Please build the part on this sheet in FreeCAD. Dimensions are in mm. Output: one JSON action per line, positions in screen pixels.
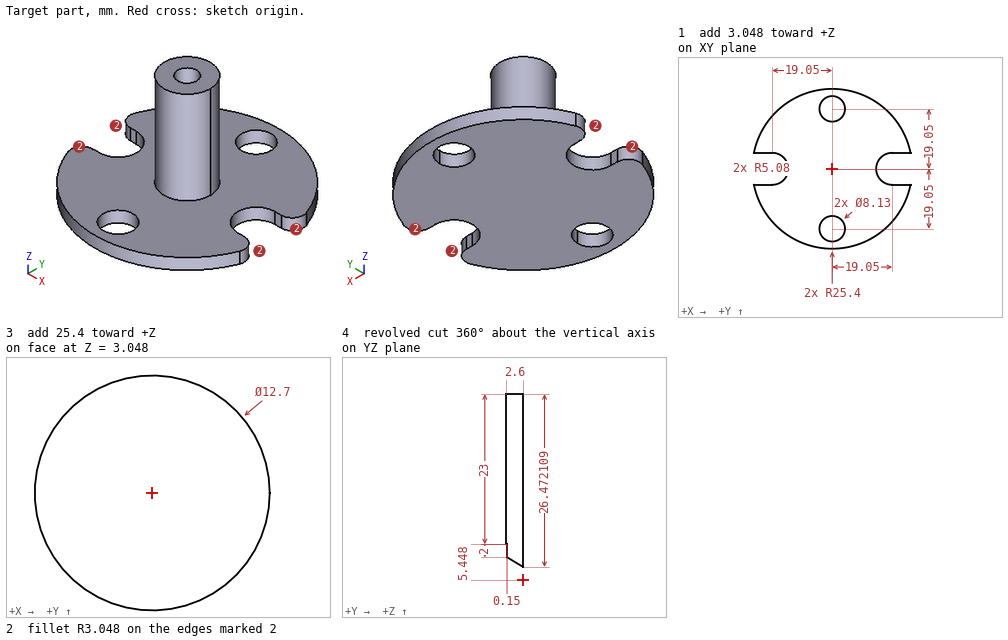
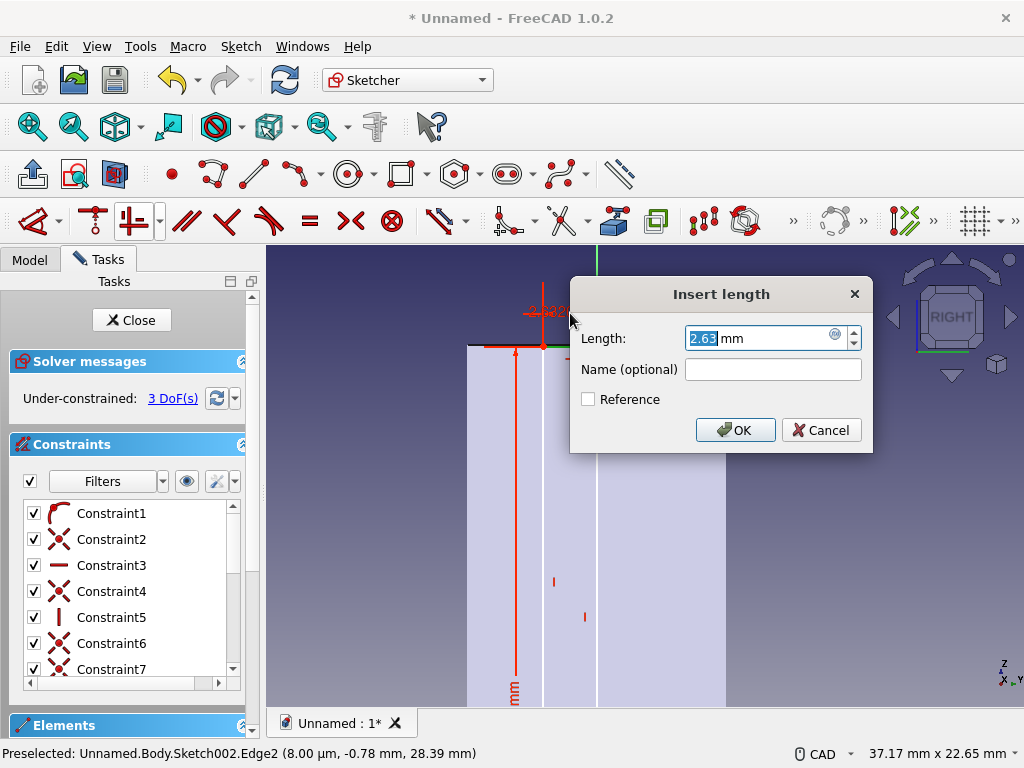
{"action": "type", "text": "2.6"}
{"action": "key", "text": "Return"}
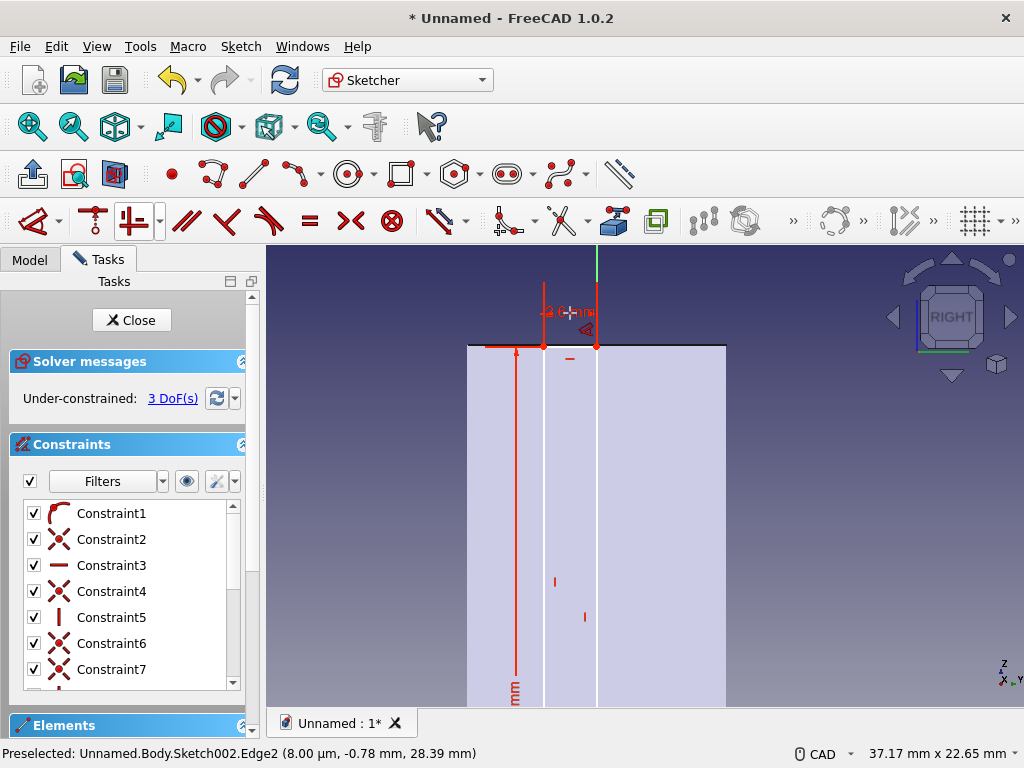
{"action": "scroll", "coordinate": [581, 346], "scroll_direction": "down", "scroll_amount": 4}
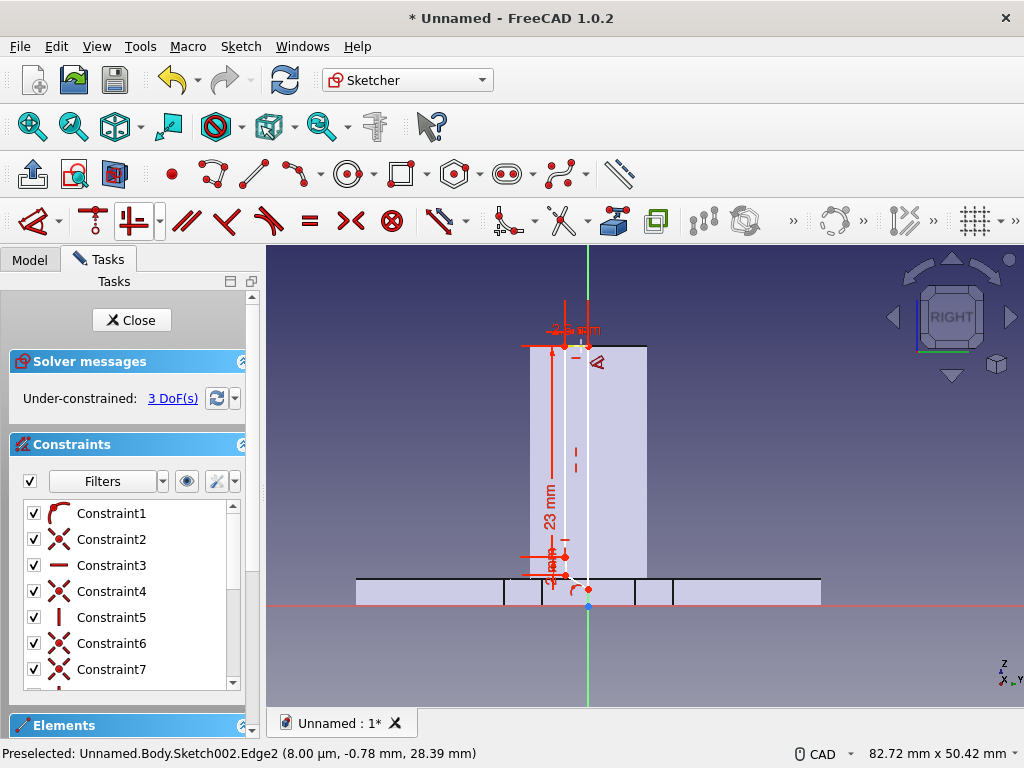
{"action": "scroll", "coordinate": [565, 557], "scroll_direction": "up", "scroll_amount": 17}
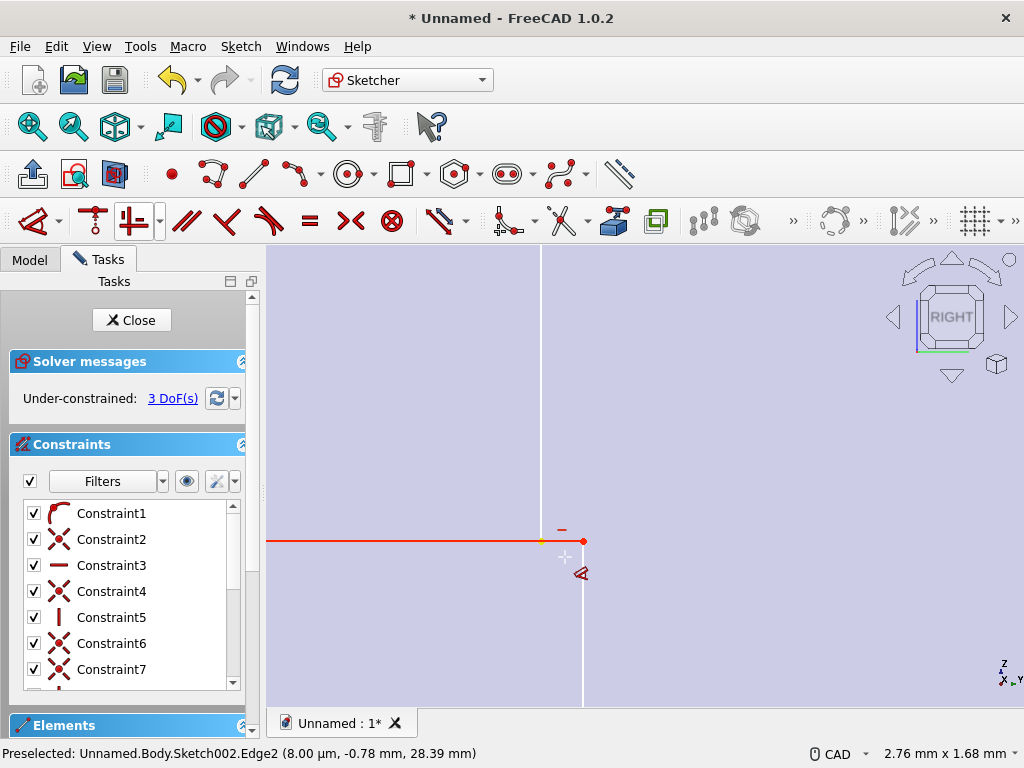
{"action": "left_click", "coordinate": [562, 541]}
{"action": "left_click", "coordinate": [562, 575]}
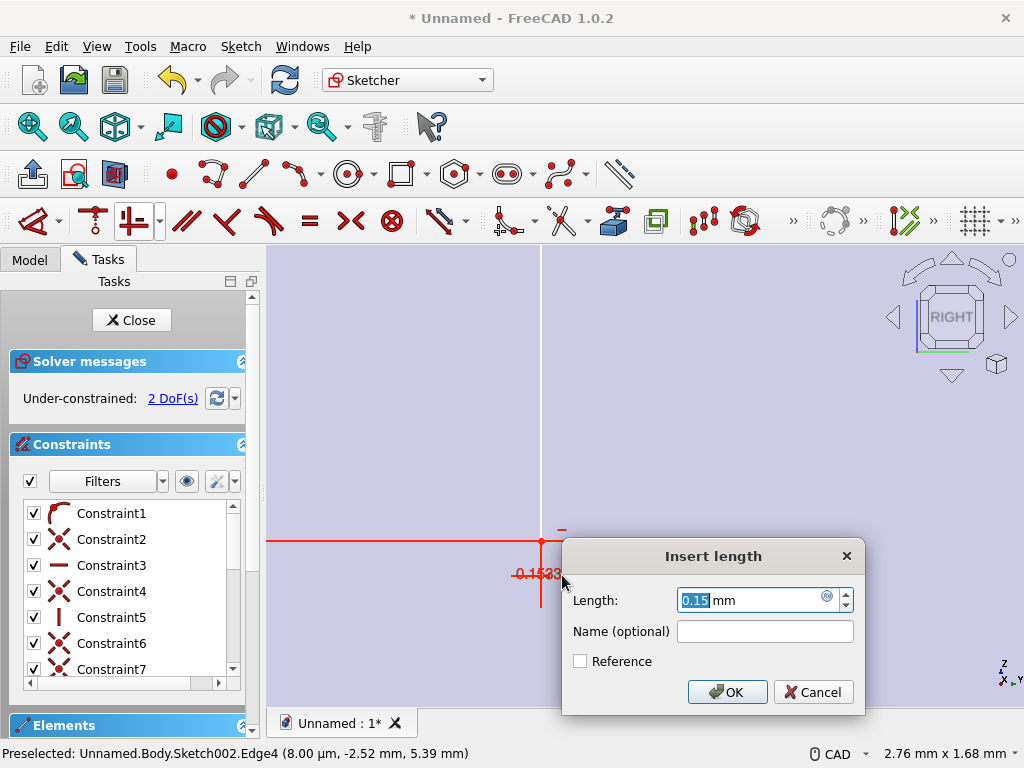
{"action": "type", "text": "0.15"}
{"action": "key", "text": "Return"}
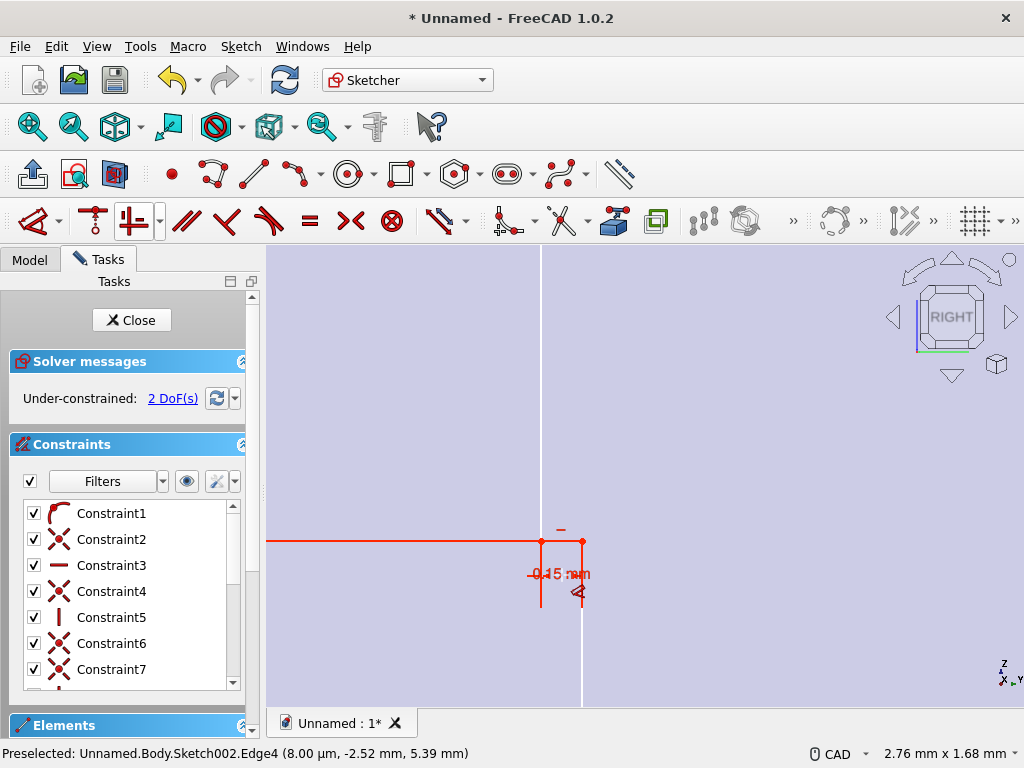
{"action": "scroll", "coordinate": [563, 576], "scroll_direction": "down", "scroll_amount": 16}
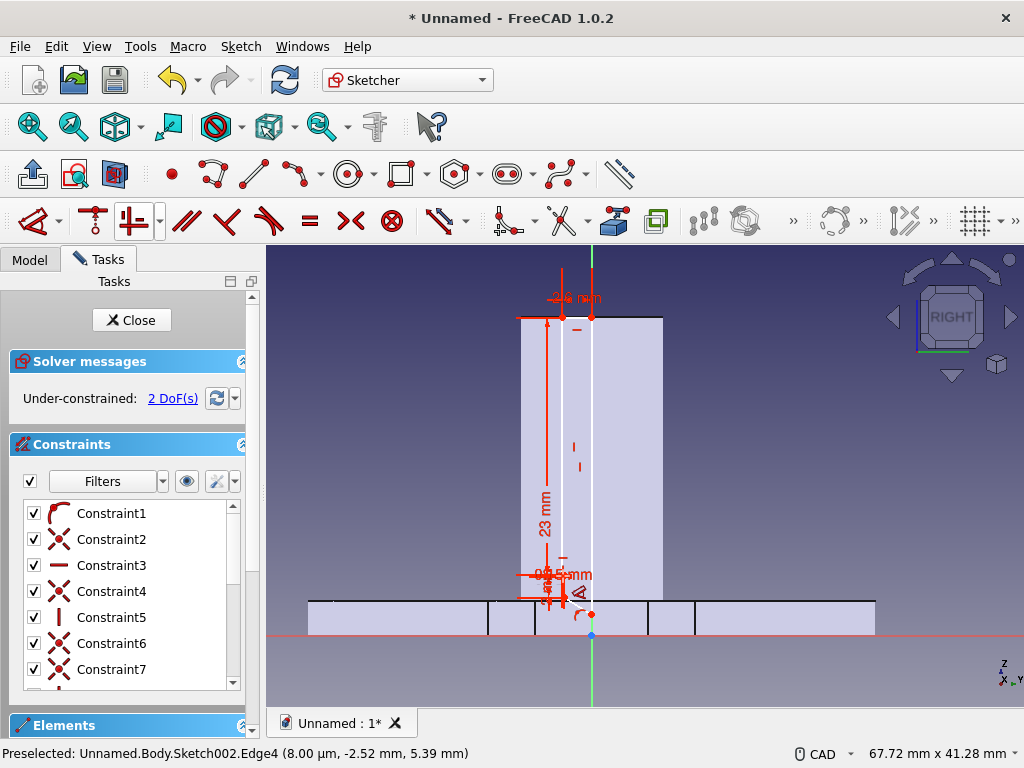
{"action": "scroll", "coordinate": [562, 575], "scroll_direction": "up", "scroll_amount": 10}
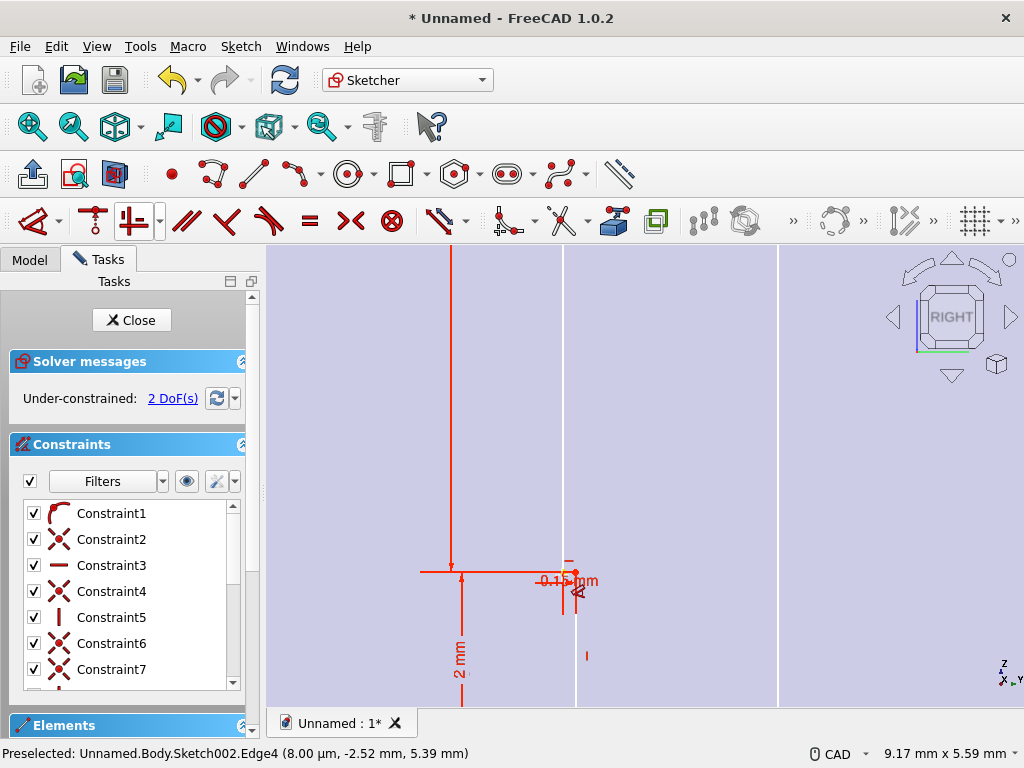
{"action": "left_click", "coordinate": [563, 572]}
{"action": "left_click", "coordinate": [812, 626]}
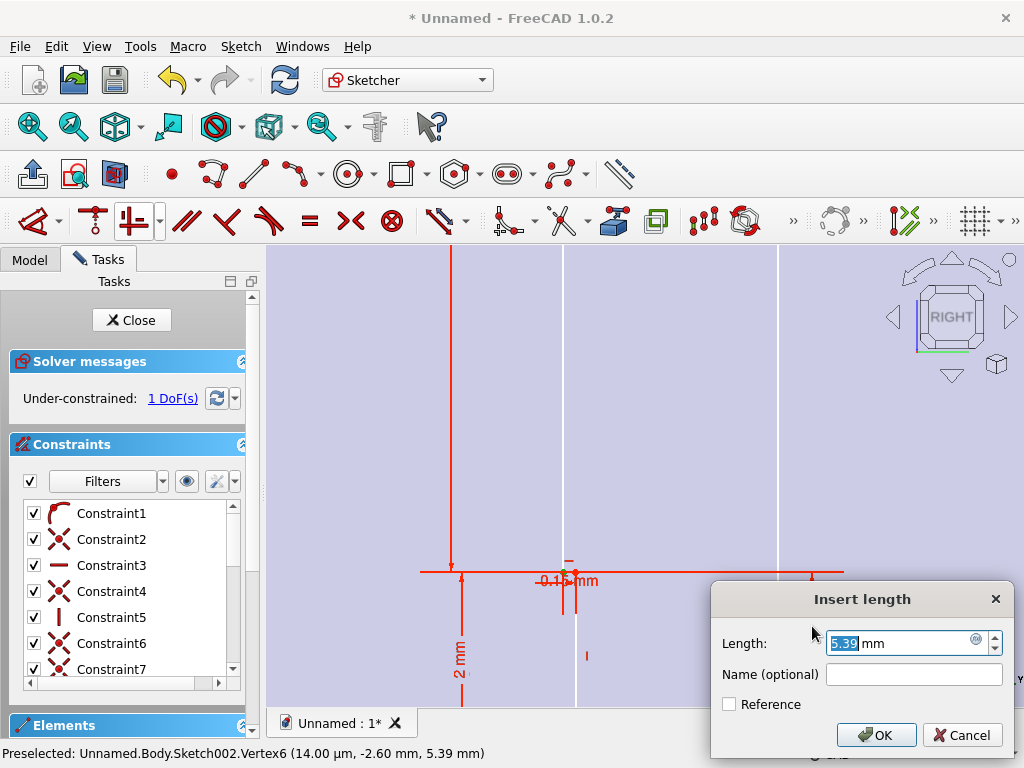
{"action": "type", "text": "5.448"}
{"action": "key", "text": "Return"}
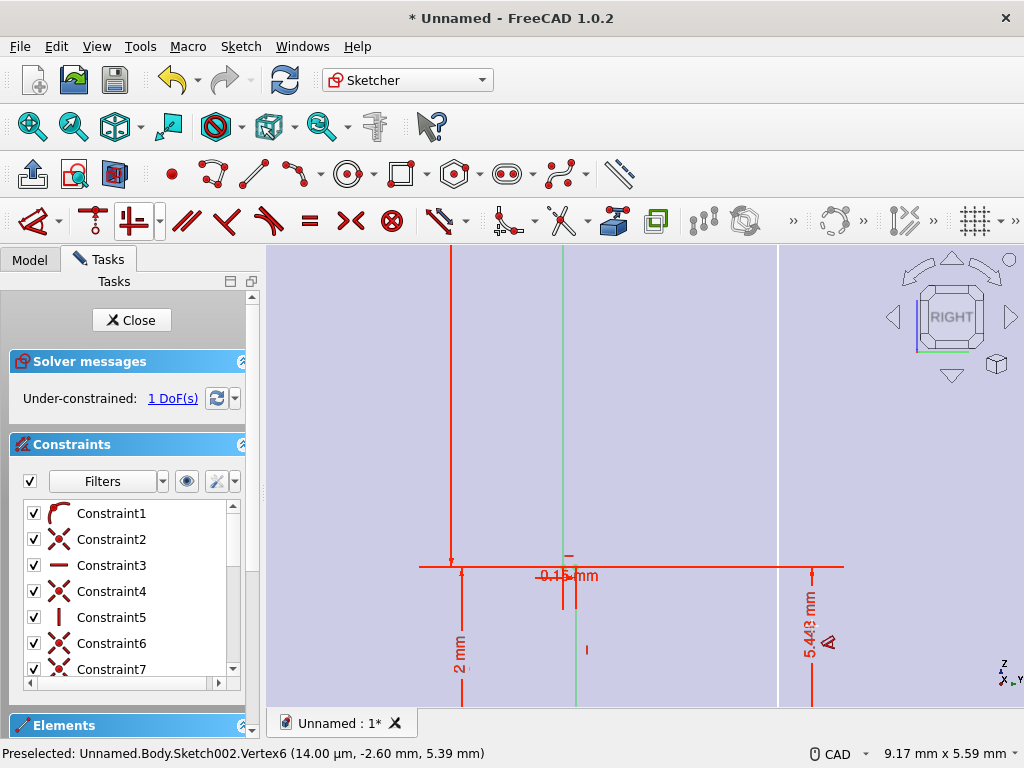
{"action": "scroll", "coordinate": [565, 555], "scroll_direction": "down", "scroll_amount": 11}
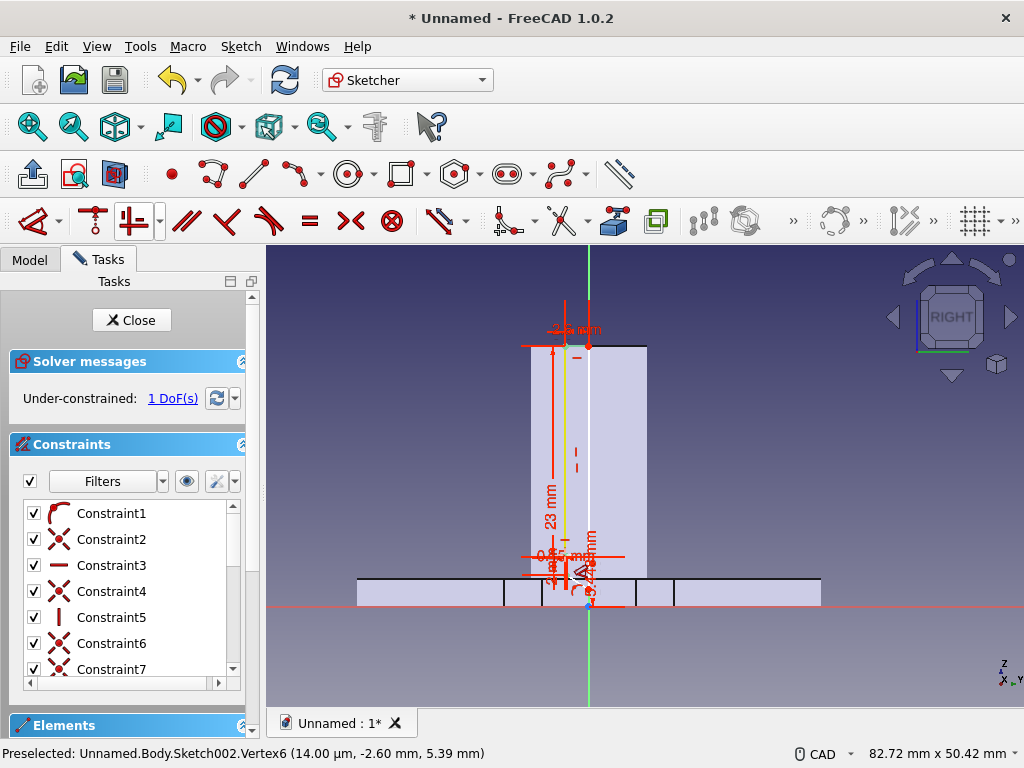
{"action": "left_click", "coordinate": [589, 541]}
{"action": "left_click", "coordinate": [623, 468]}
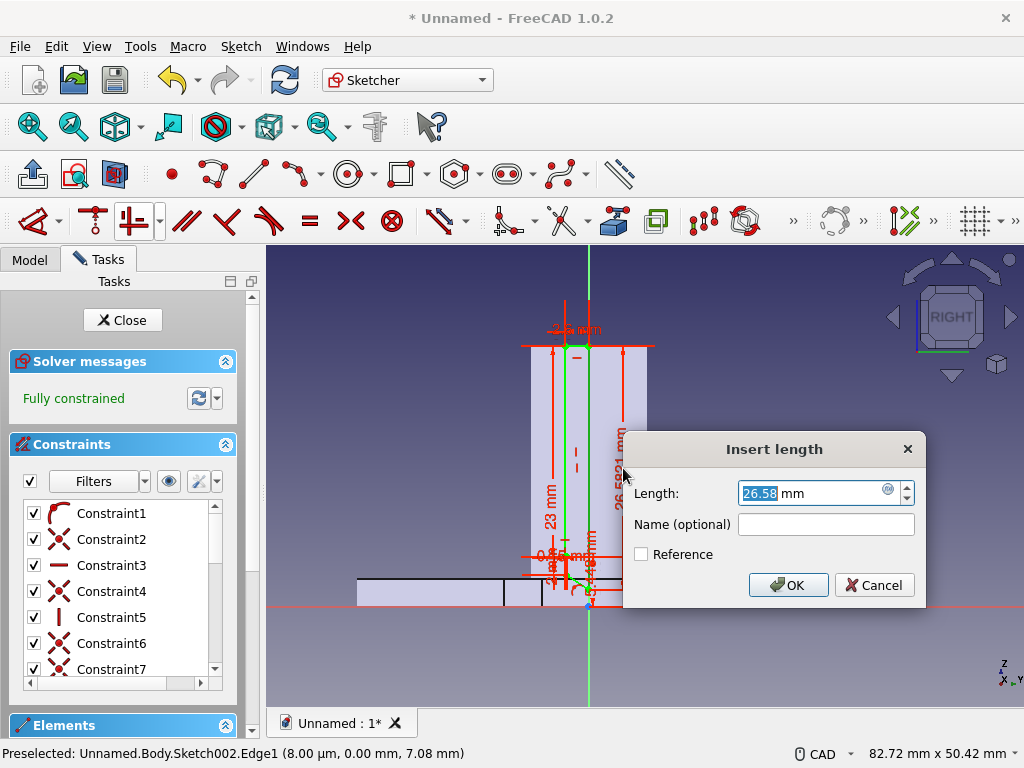
{"action": "type", "text": "26.472109"}
{"action": "key", "text": "Return"}
{"action": "key", "text": "Escape"}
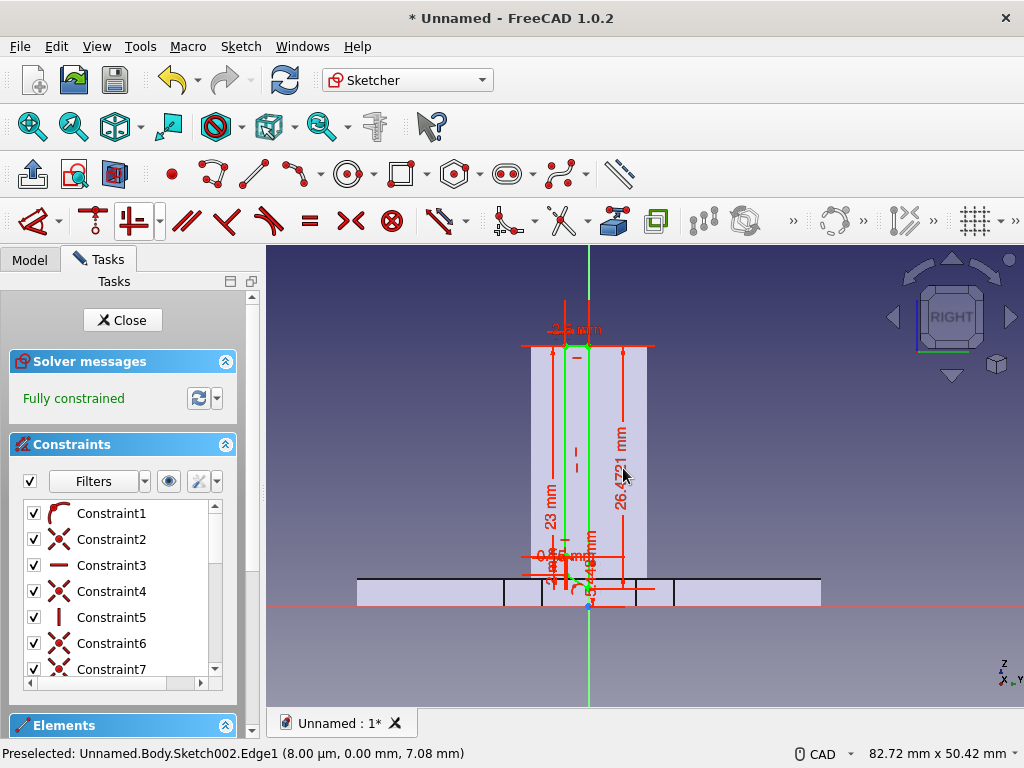
{"action": "left_click", "coordinate": [123, 320]}